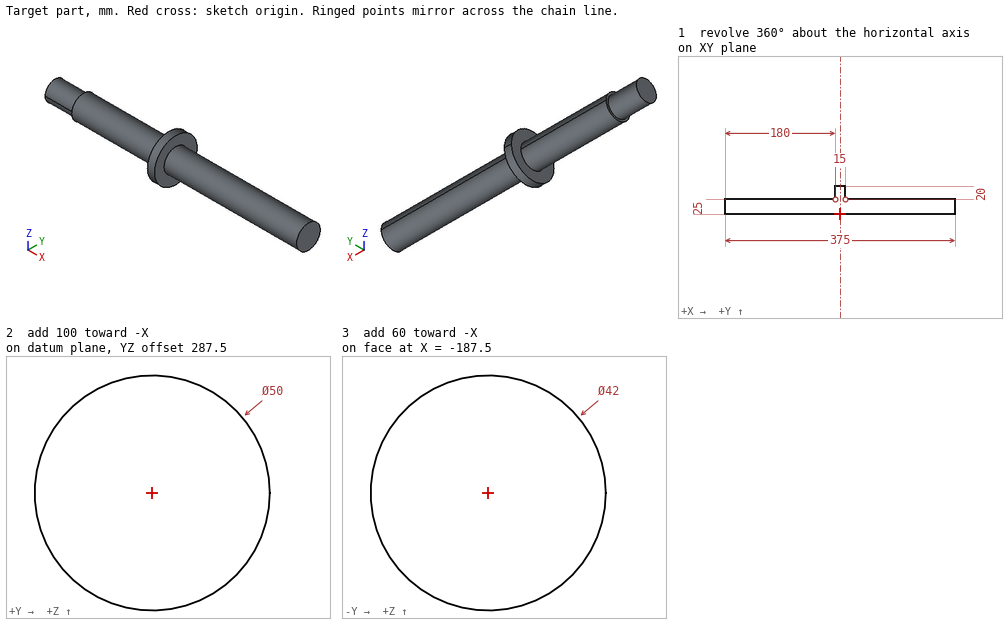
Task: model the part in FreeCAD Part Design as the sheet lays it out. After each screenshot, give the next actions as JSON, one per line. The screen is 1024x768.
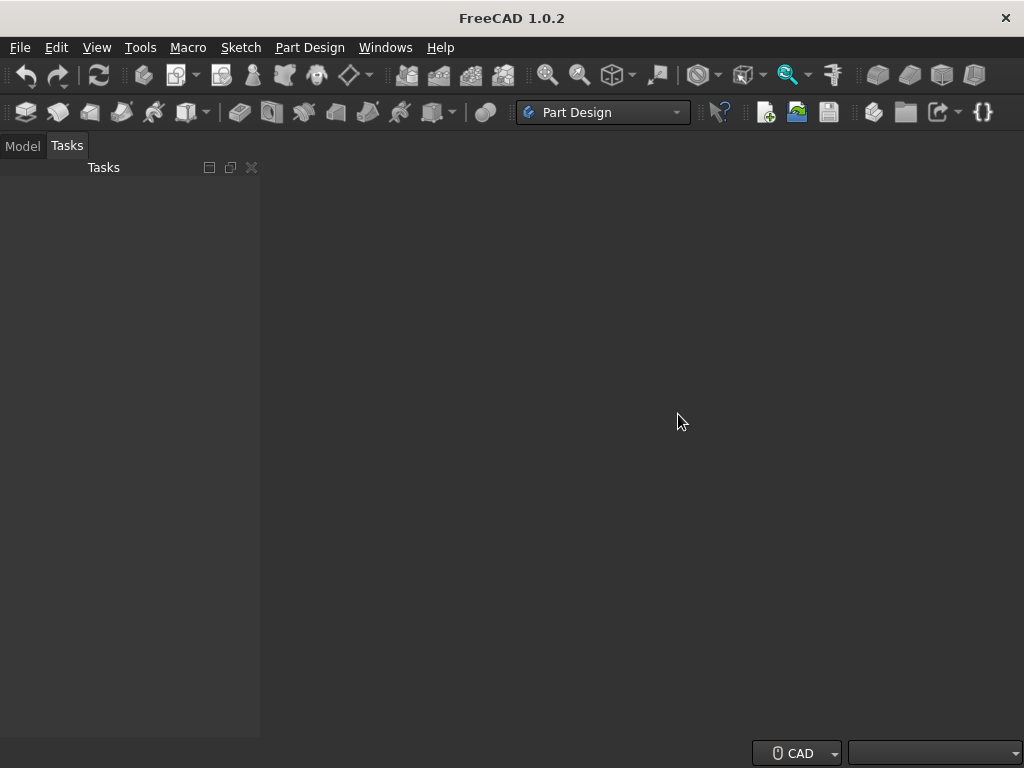
{"action": "left_click", "coordinate": [766, 112]}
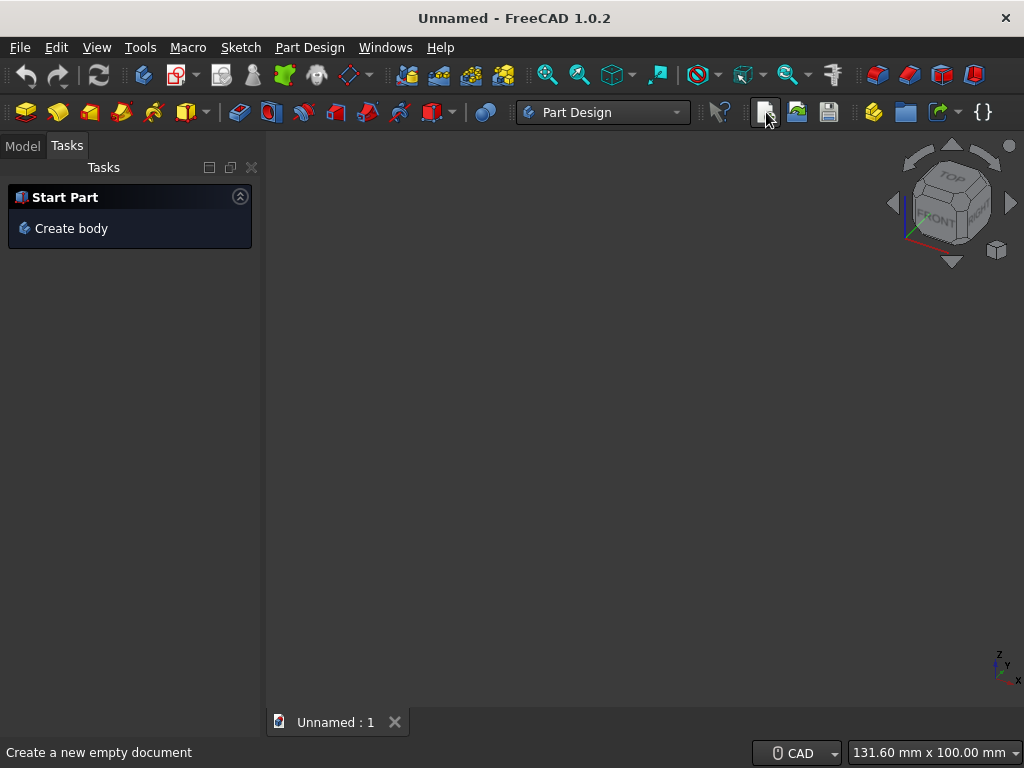
{"action": "left_click", "coordinate": [176, 76]}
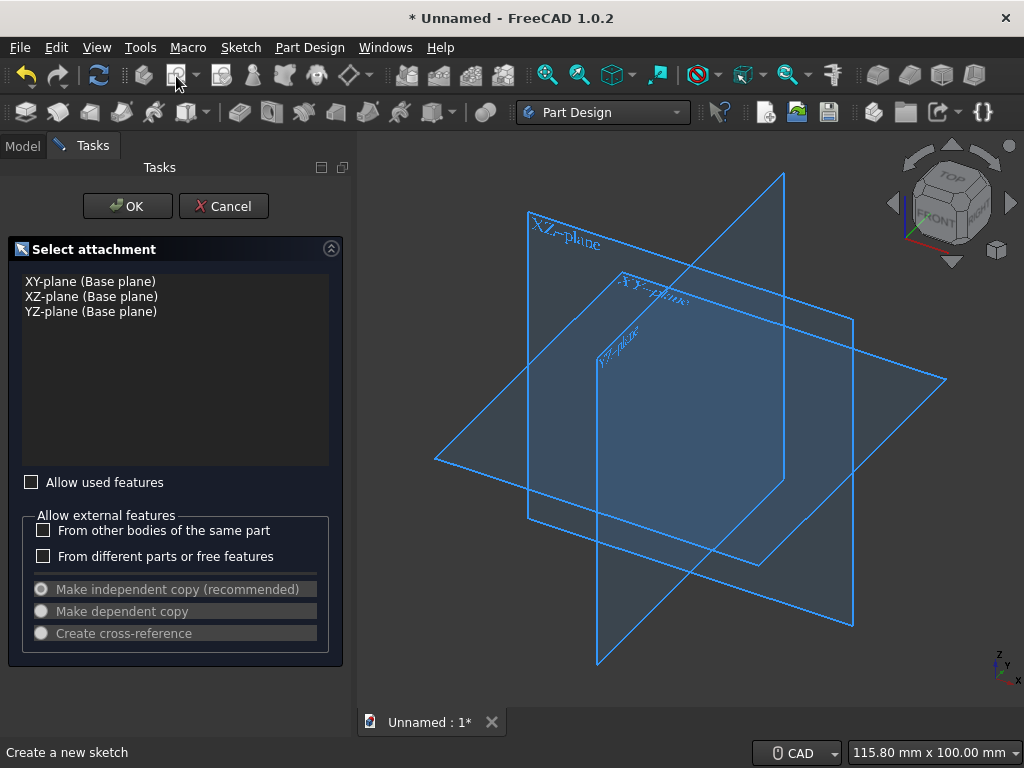
{"action": "left_click", "coordinate": [82, 282]}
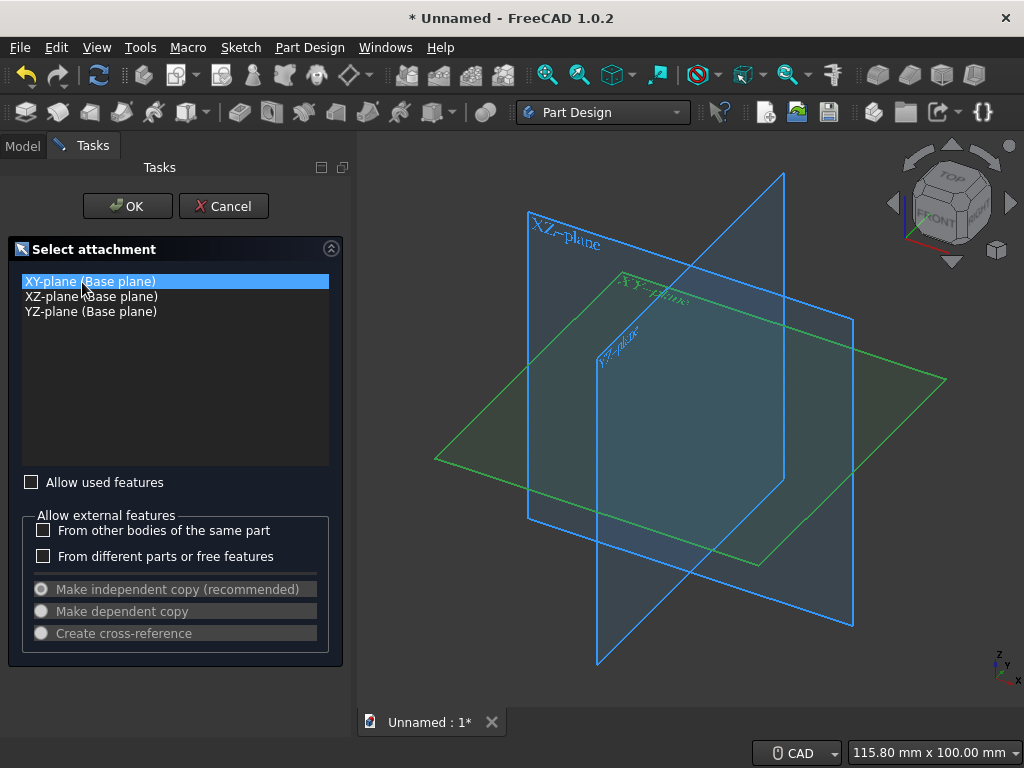
{"action": "left_click", "coordinate": [128, 206]}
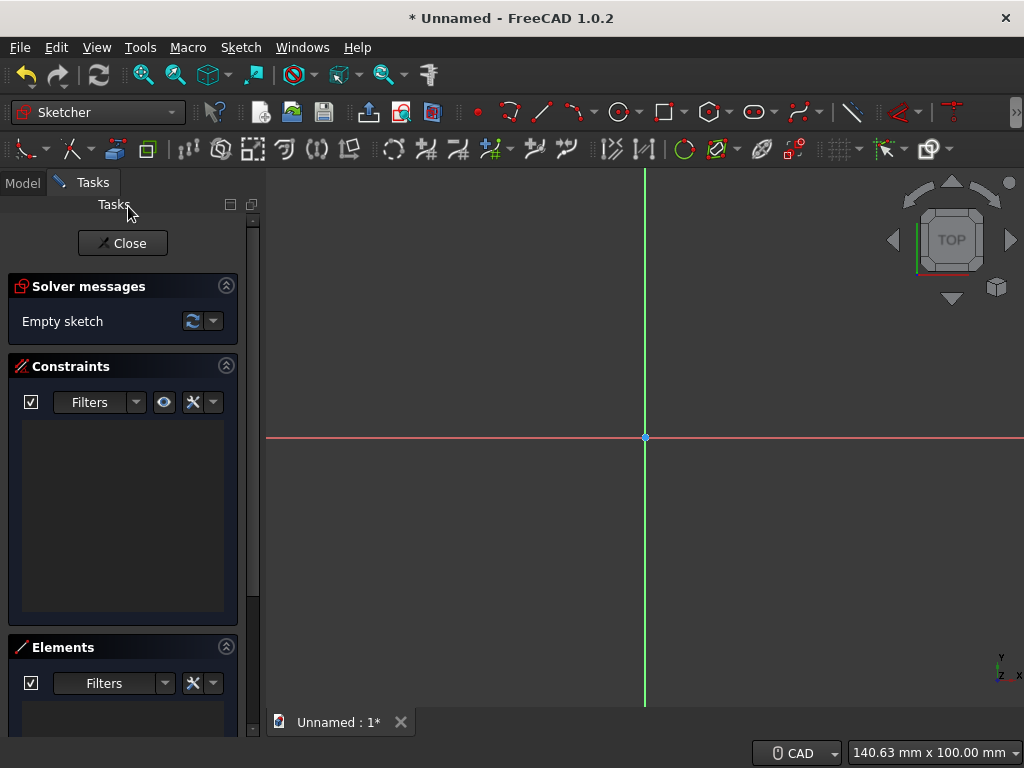
{"action": "scroll", "coordinate": [559, 468], "scroll_direction": "down", "scroll_amount": 8}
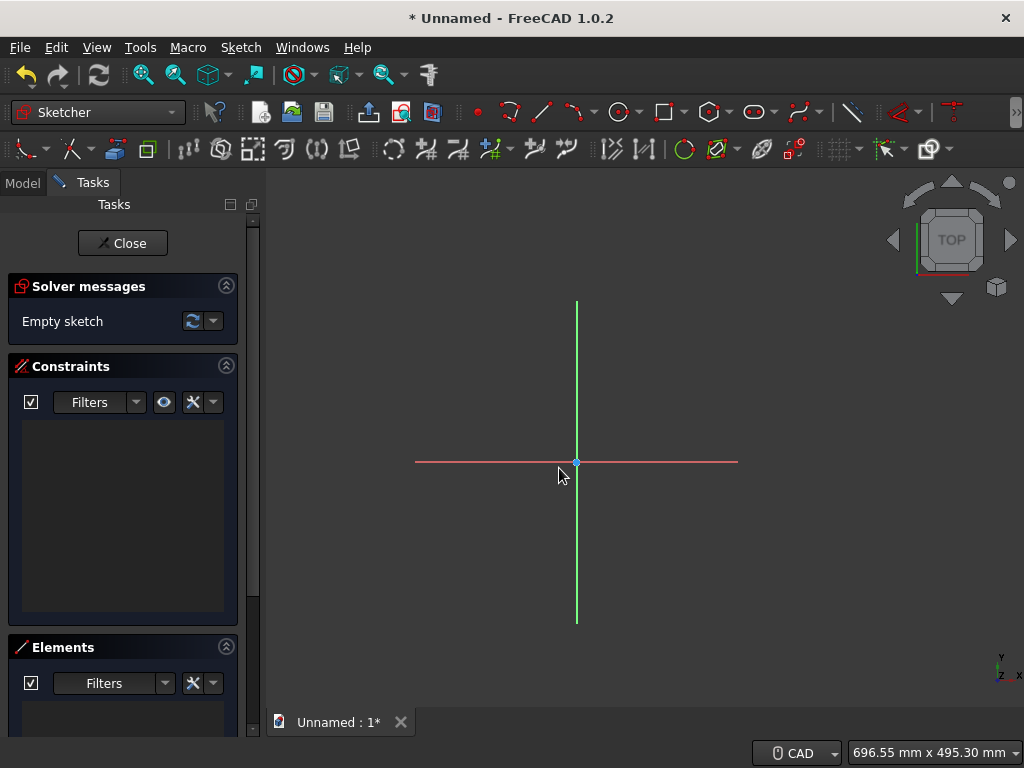
{"action": "left_click", "coordinate": [510, 112]}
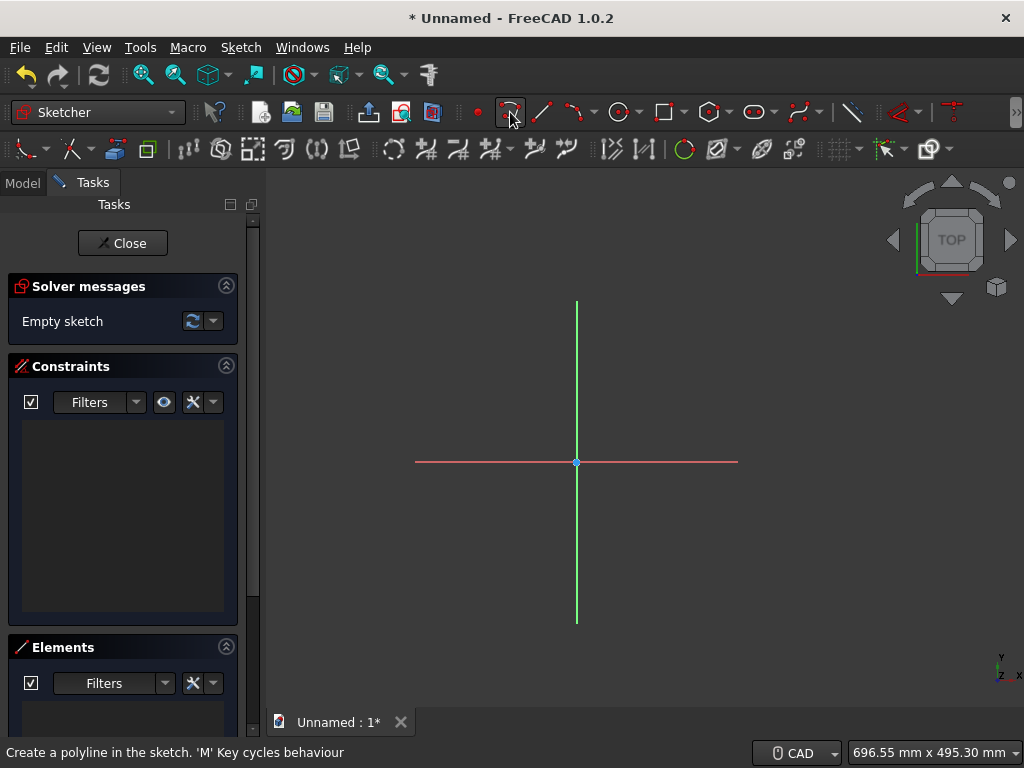
{"action": "scroll", "coordinate": [585, 435], "scroll_direction": "up", "scroll_amount": 4}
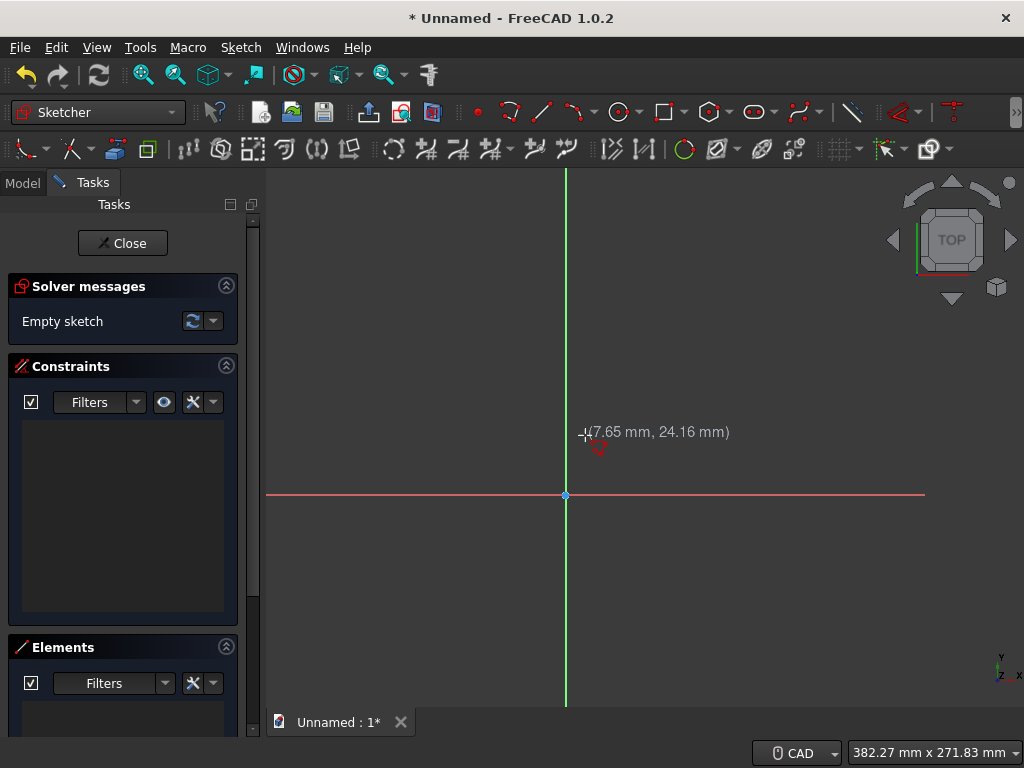
{"action": "left_click", "coordinate": [584, 435]}
{"action": "left_click", "coordinate": [584, 386]}
{"action": "left_click", "coordinate": [548, 386]}
{"action": "left_click", "coordinate": [548, 435]}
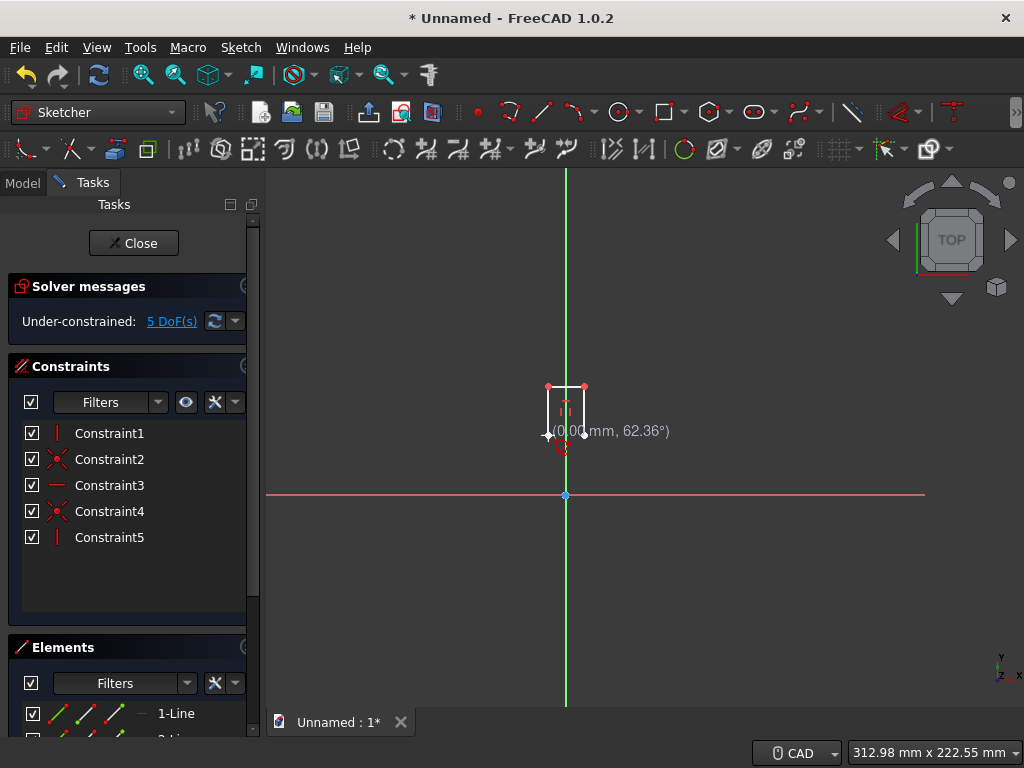
{"action": "scroll", "coordinate": [585, 435], "scroll_direction": "down", "scroll_amount": 4}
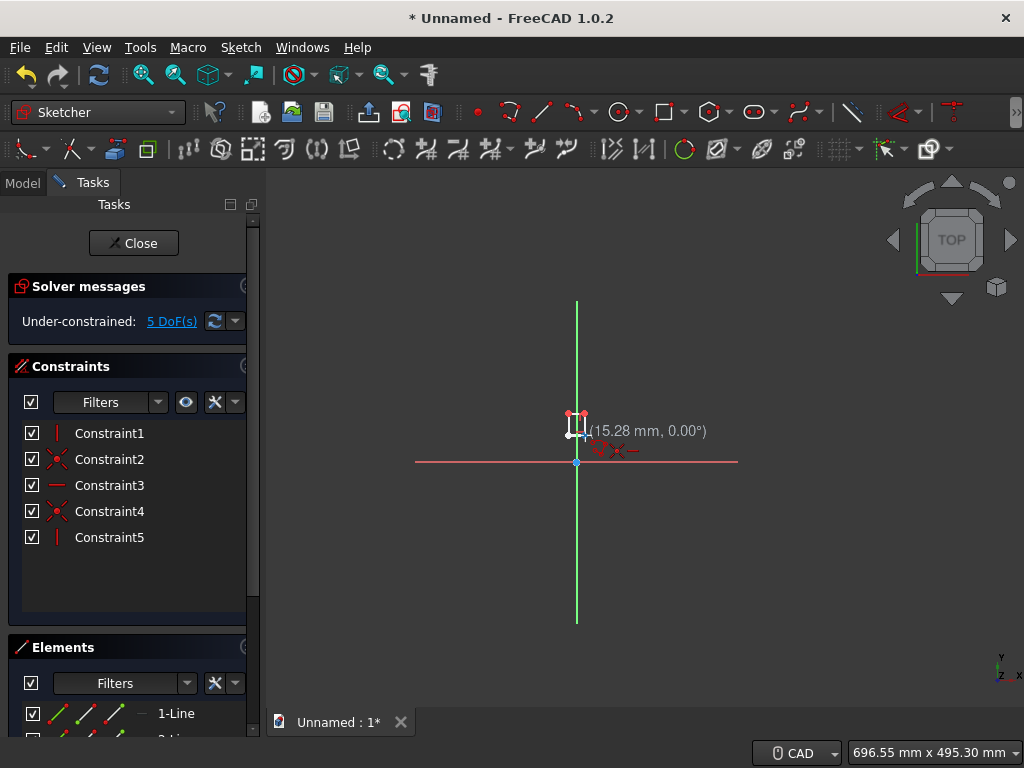
{"action": "left_click", "coordinate": [373, 435]}
{"action": "left_click", "coordinate": [373, 462]}
{"action": "left_click", "coordinate": [781, 453]}
{"action": "left_click", "coordinate": [781, 435]}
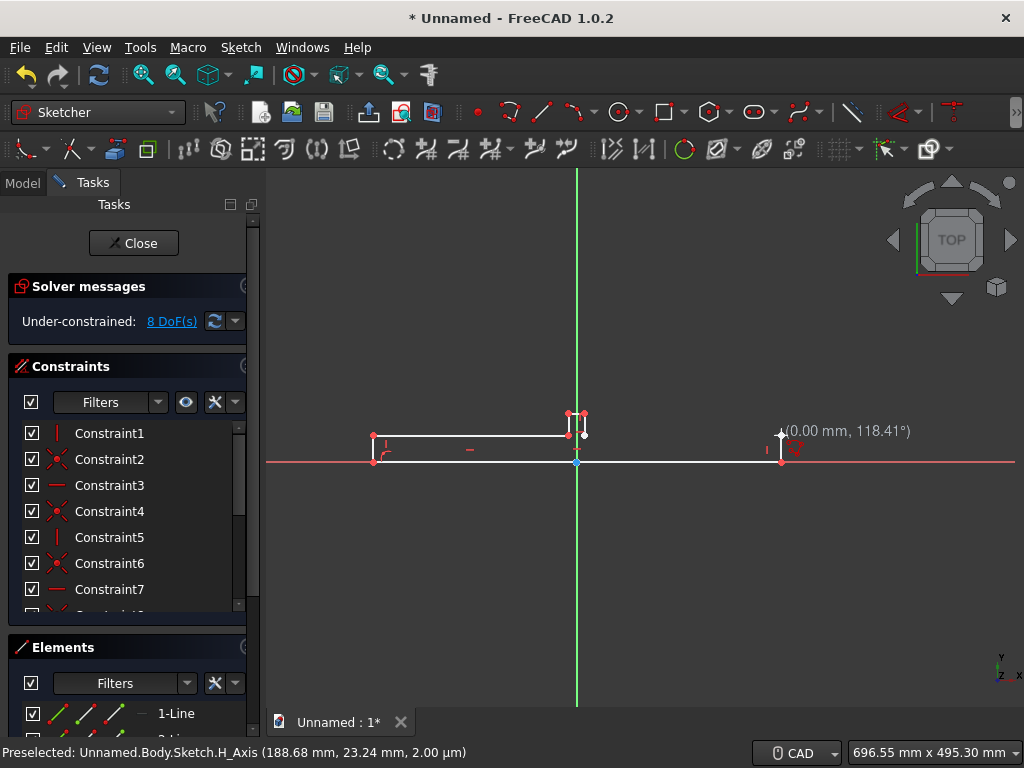
{"action": "scroll", "coordinate": [585, 435], "scroll_direction": "up", "scroll_amount": 4}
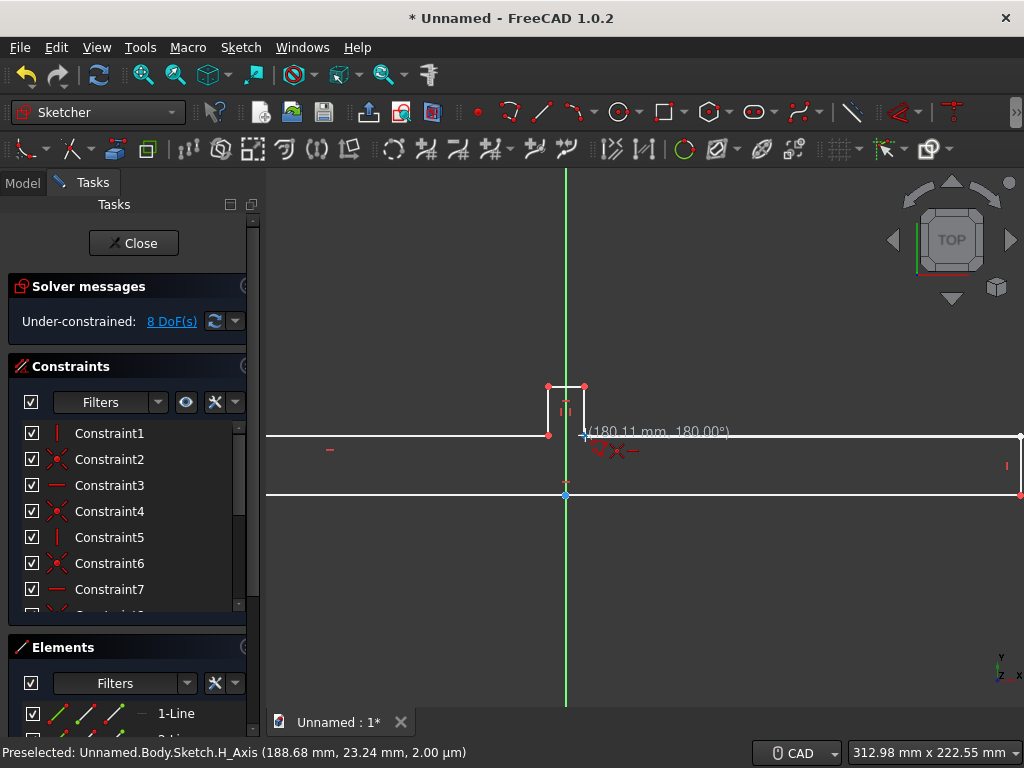
{"action": "left_click", "coordinate": [584, 436]}
{"action": "key", "text": "Escape"}
{"action": "key", "text": "Escape"}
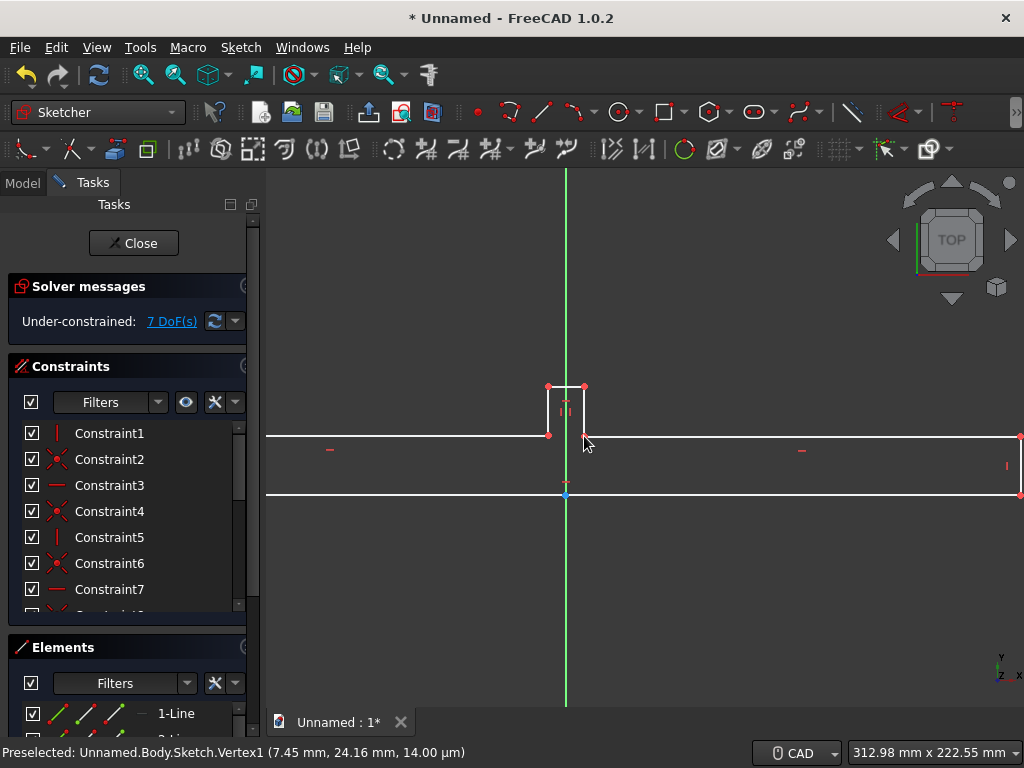
{"action": "left_click", "coordinate": [584, 437]}